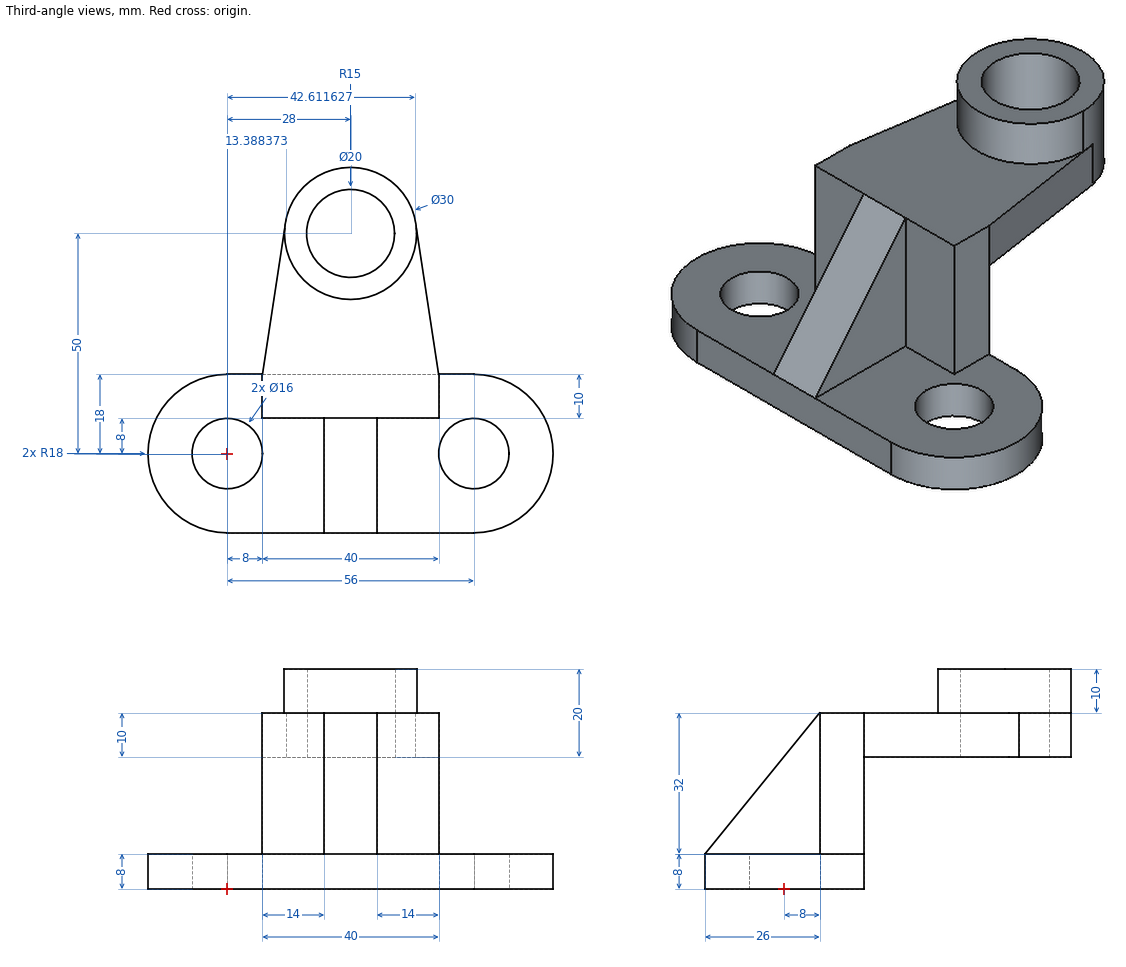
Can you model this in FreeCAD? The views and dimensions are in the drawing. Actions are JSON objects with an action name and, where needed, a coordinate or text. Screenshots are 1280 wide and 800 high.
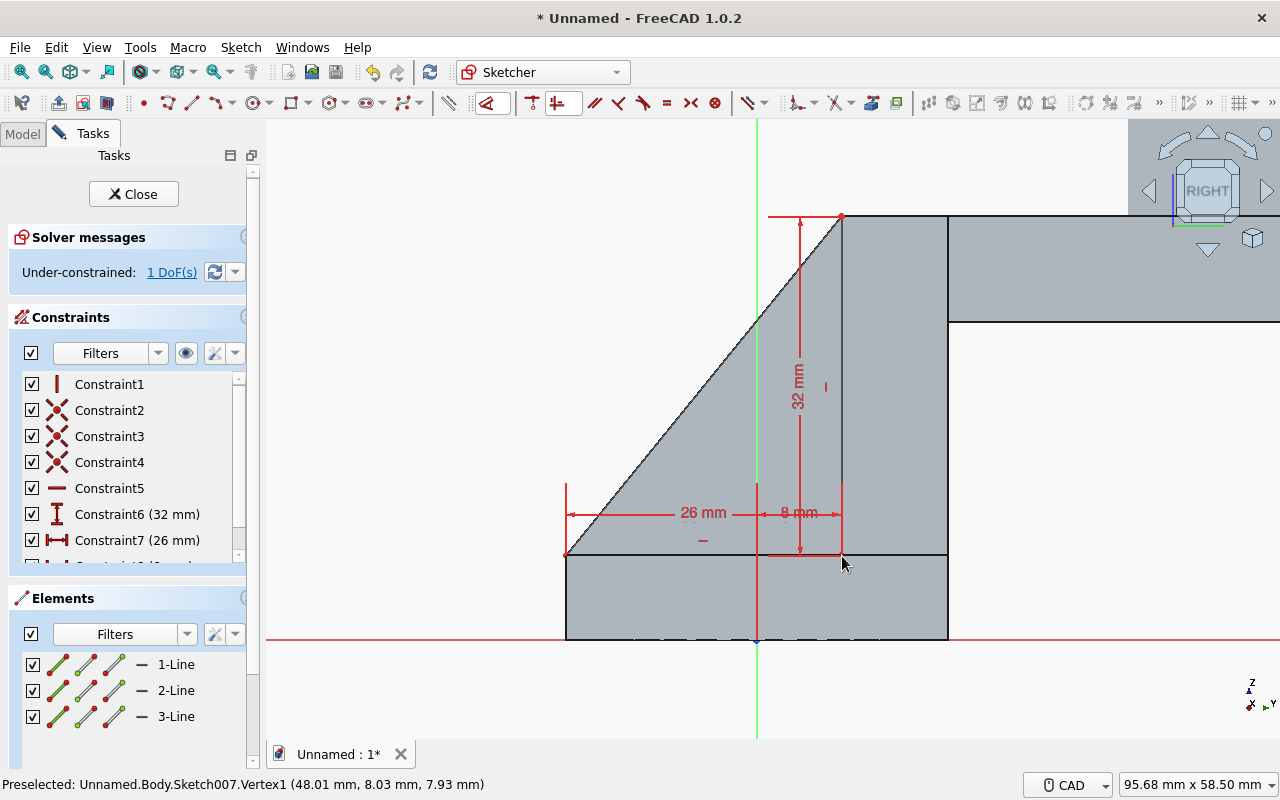
{"action": "left_click", "coordinate": [842, 556]}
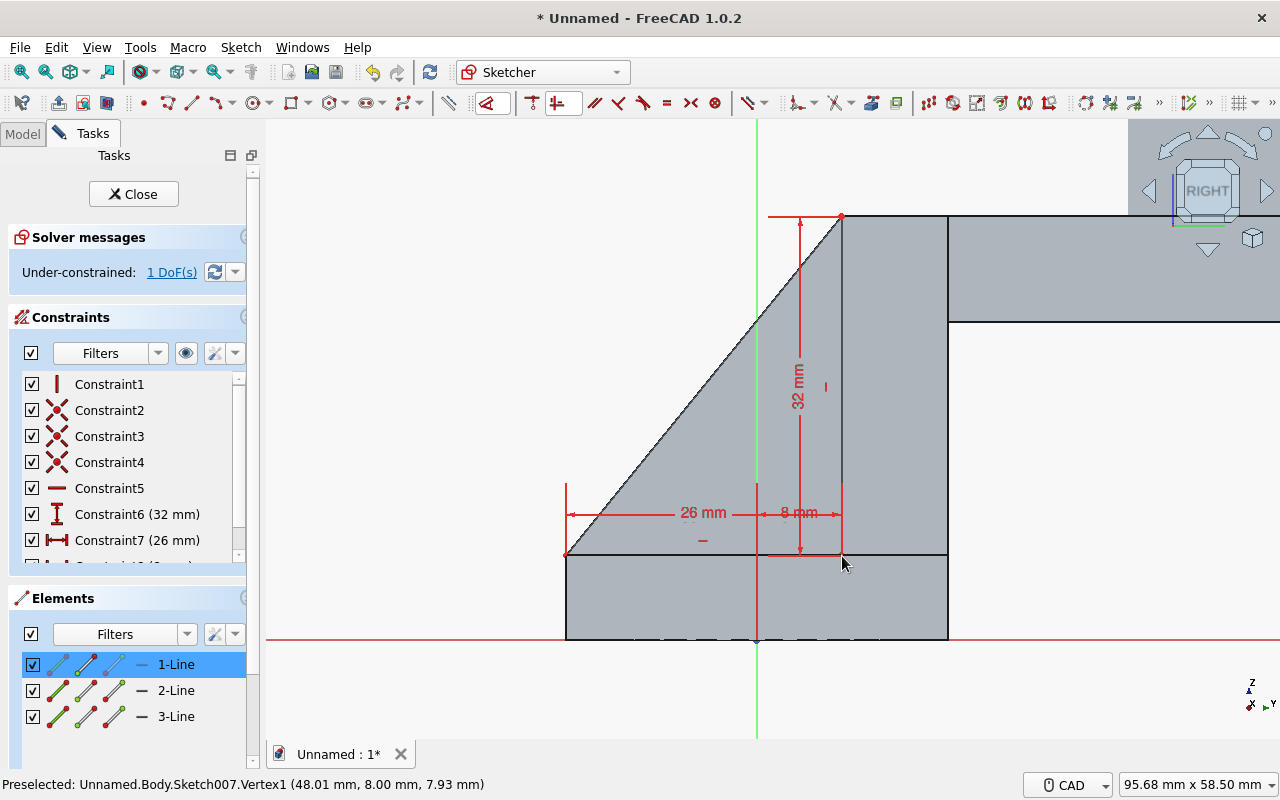
{"action": "key", "text": "i"}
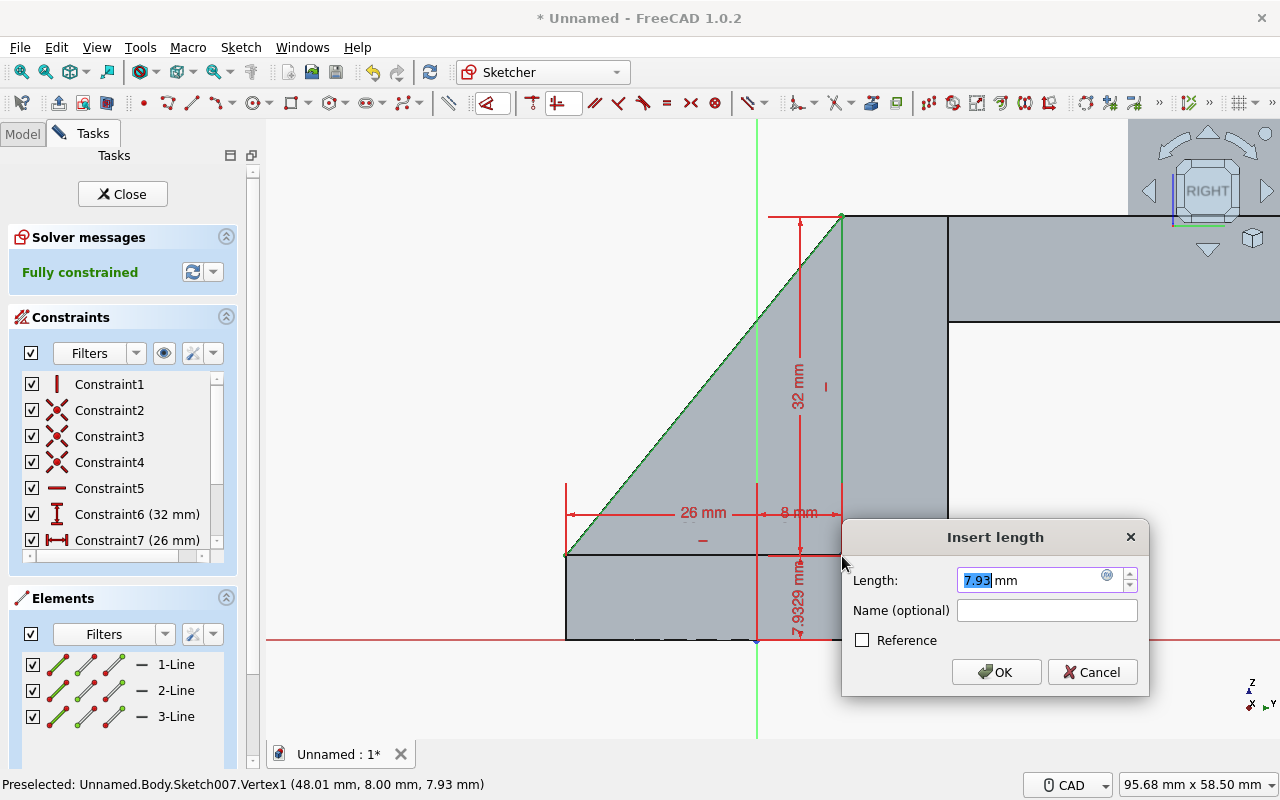
{"action": "type", "text": "8"}
{"action": "key", "text": "Return"}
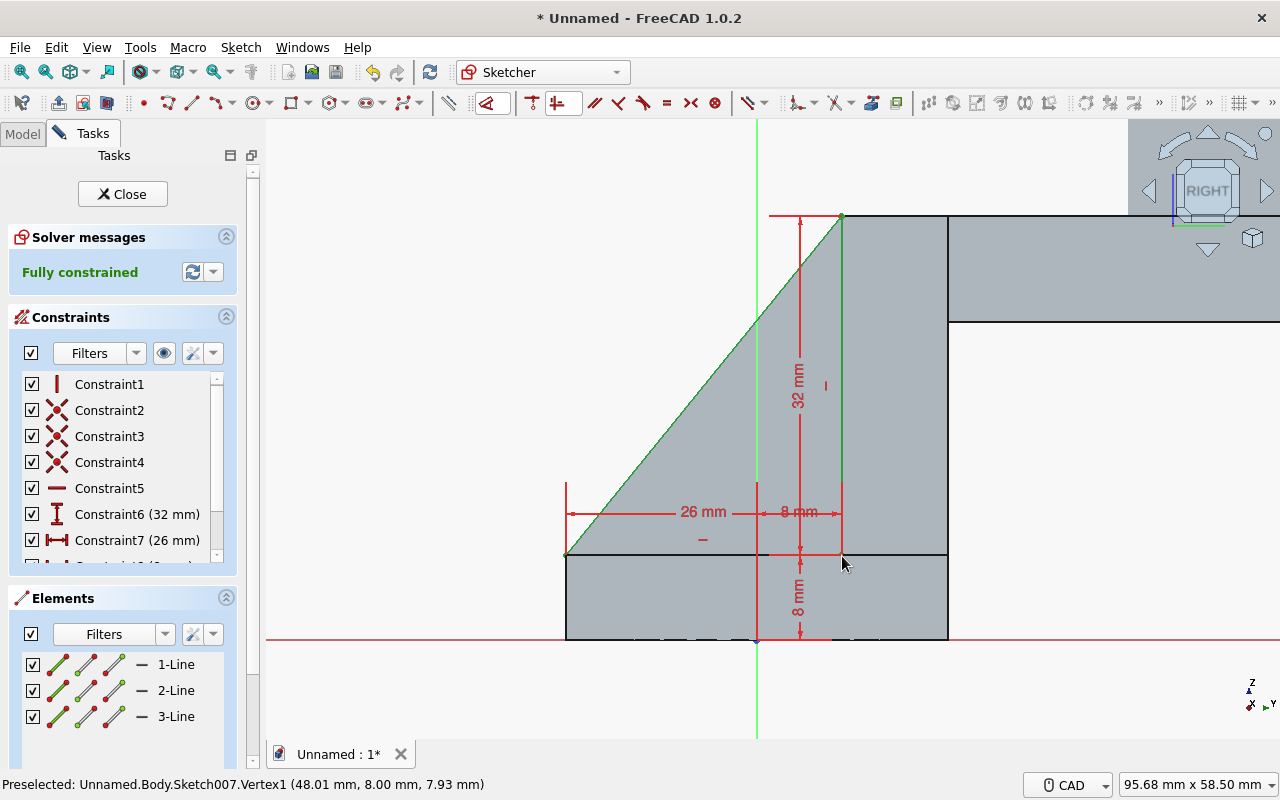
{"action": "left_click", "coordinate": [123, 194]}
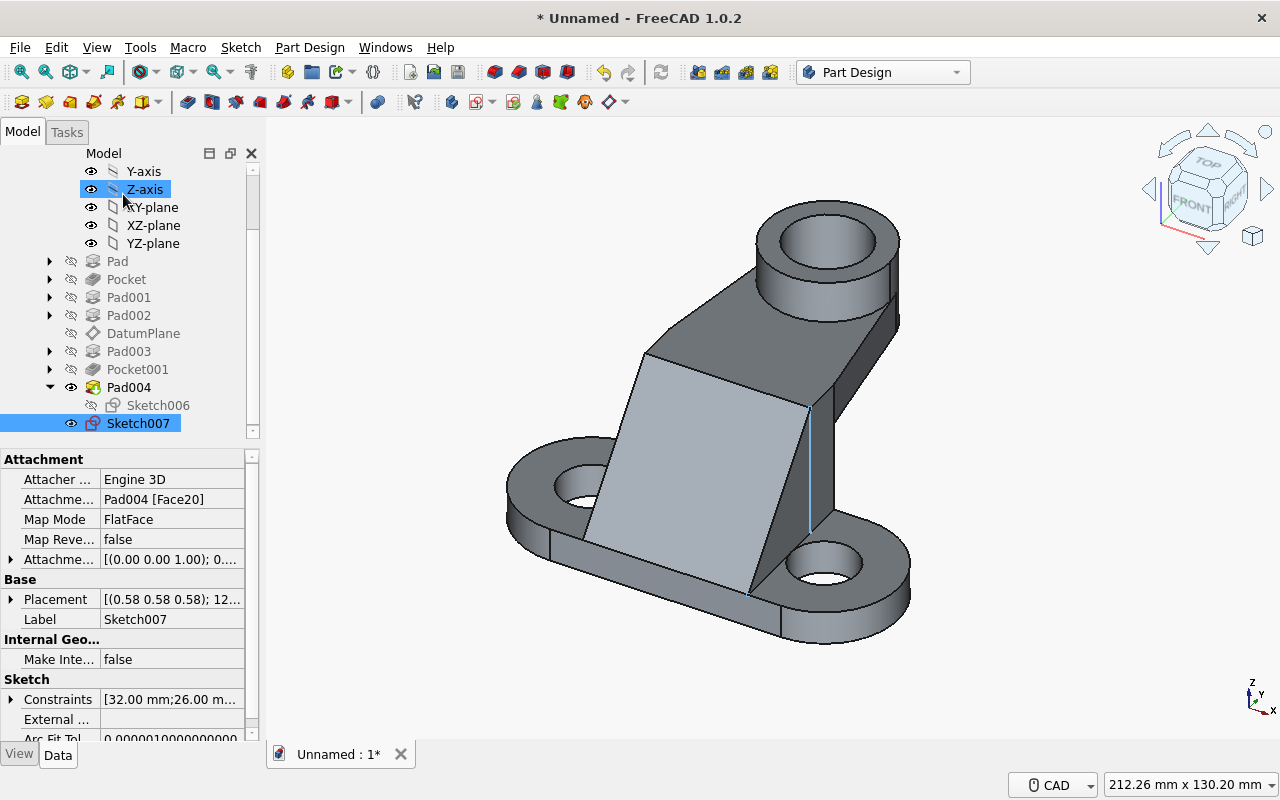
{"action": "left_click", "coordinate": [188, 102]}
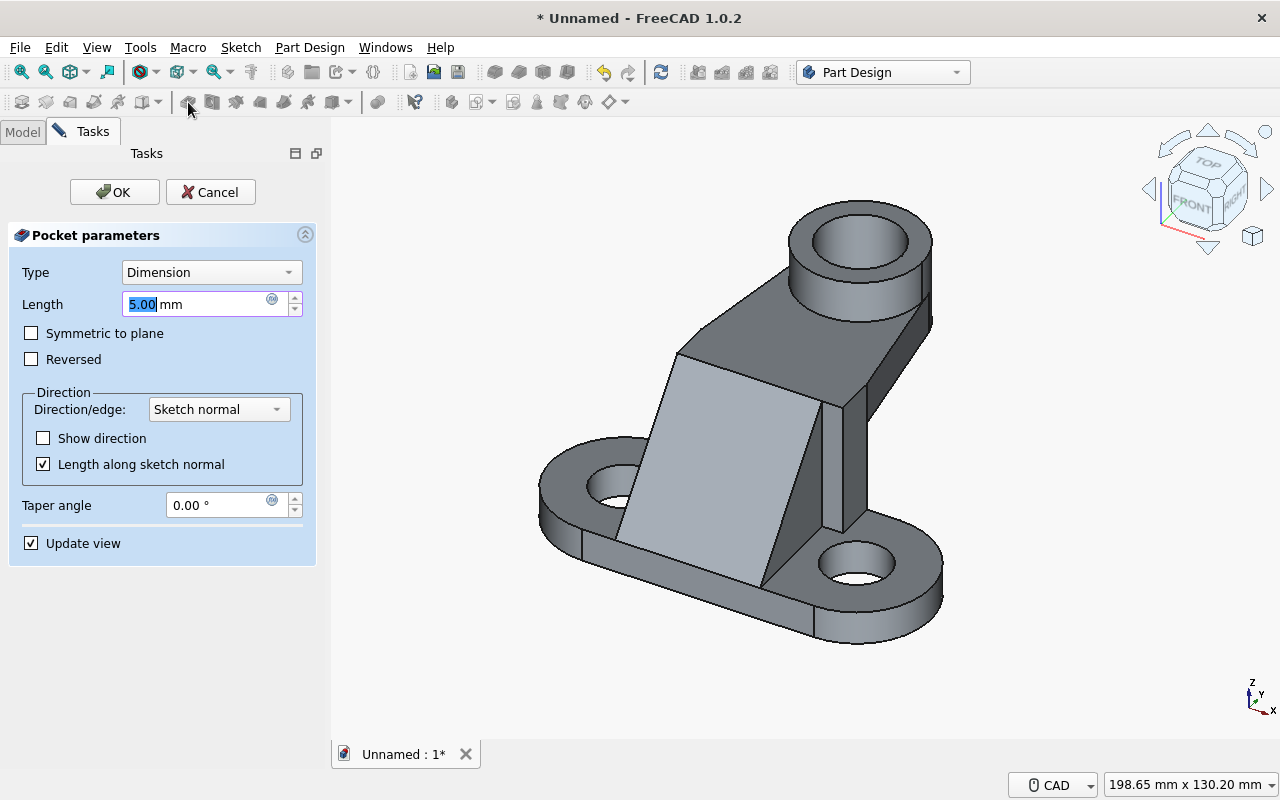
{"action": "type", "text": "14"}
{"action": "key", "text": "Tab"}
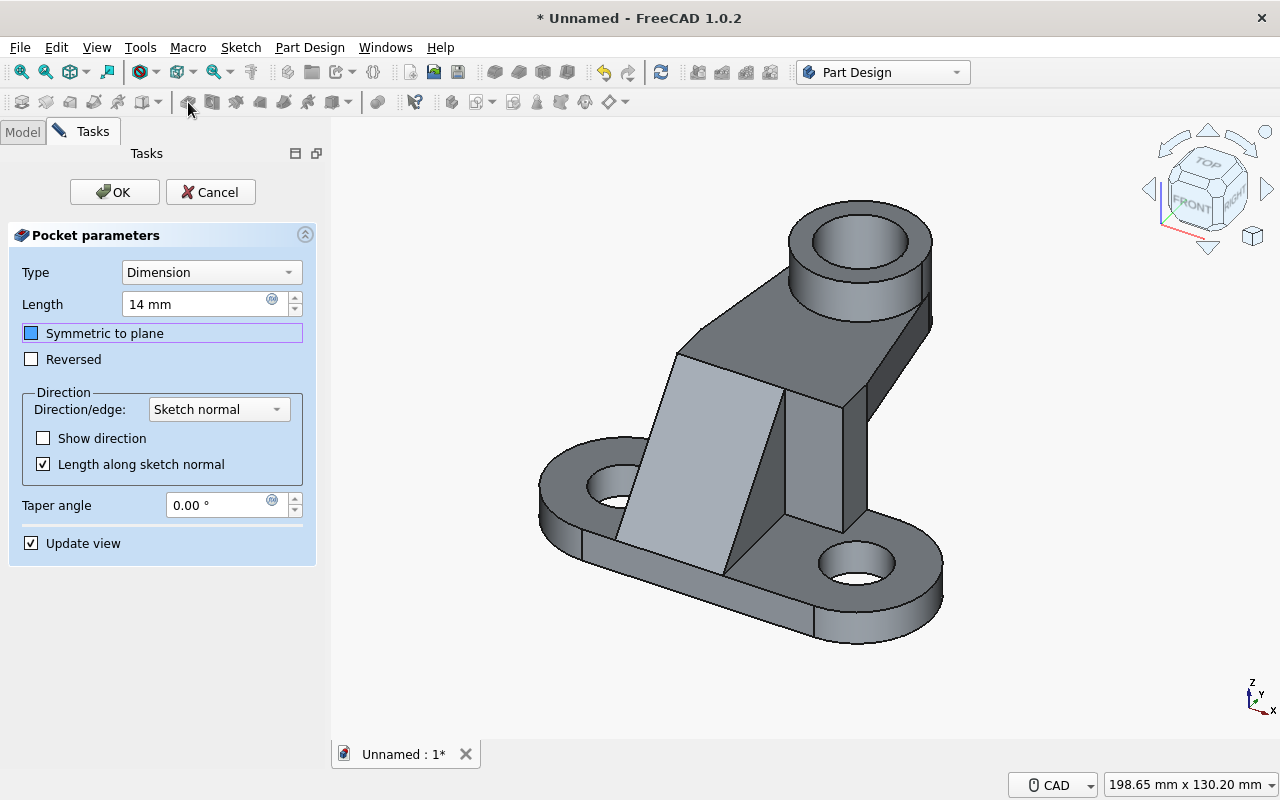
{"action": "left_click", "coordinate": [115, 192]}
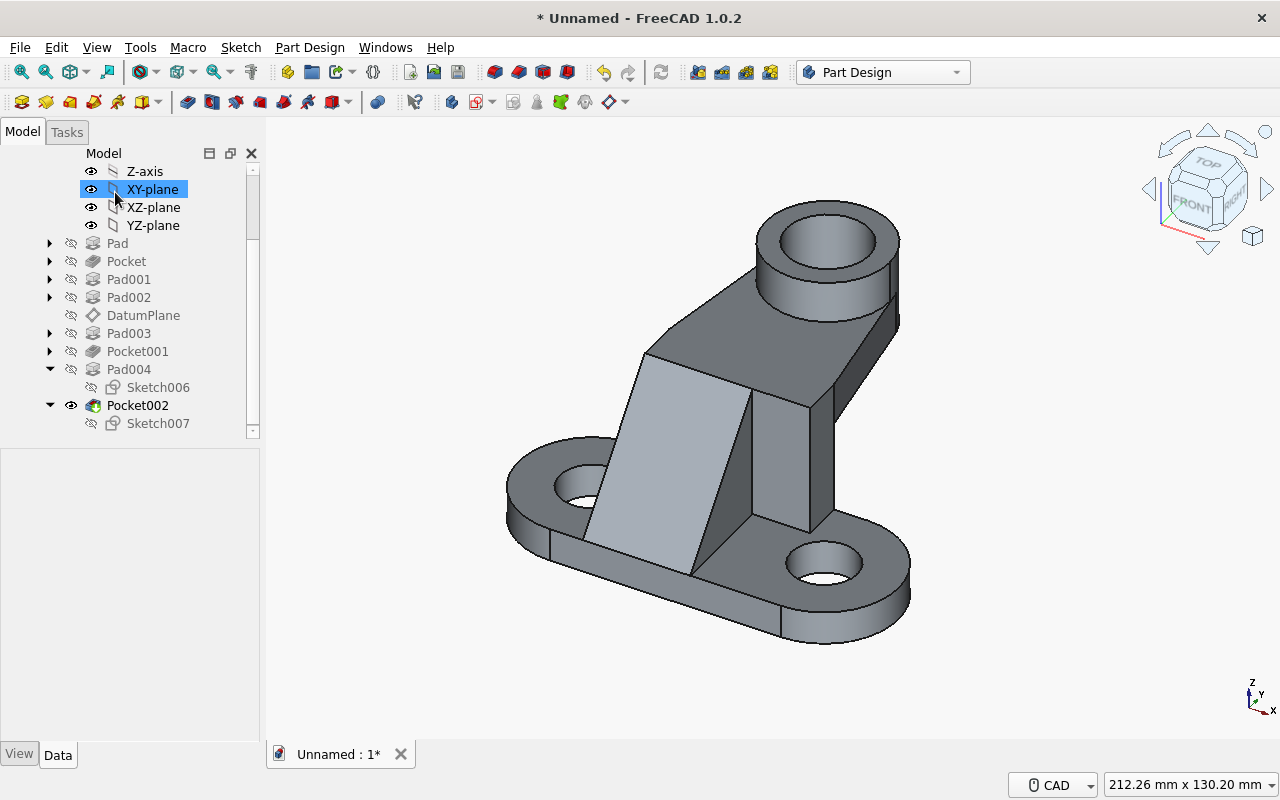
{"action": "key", "text": "6"}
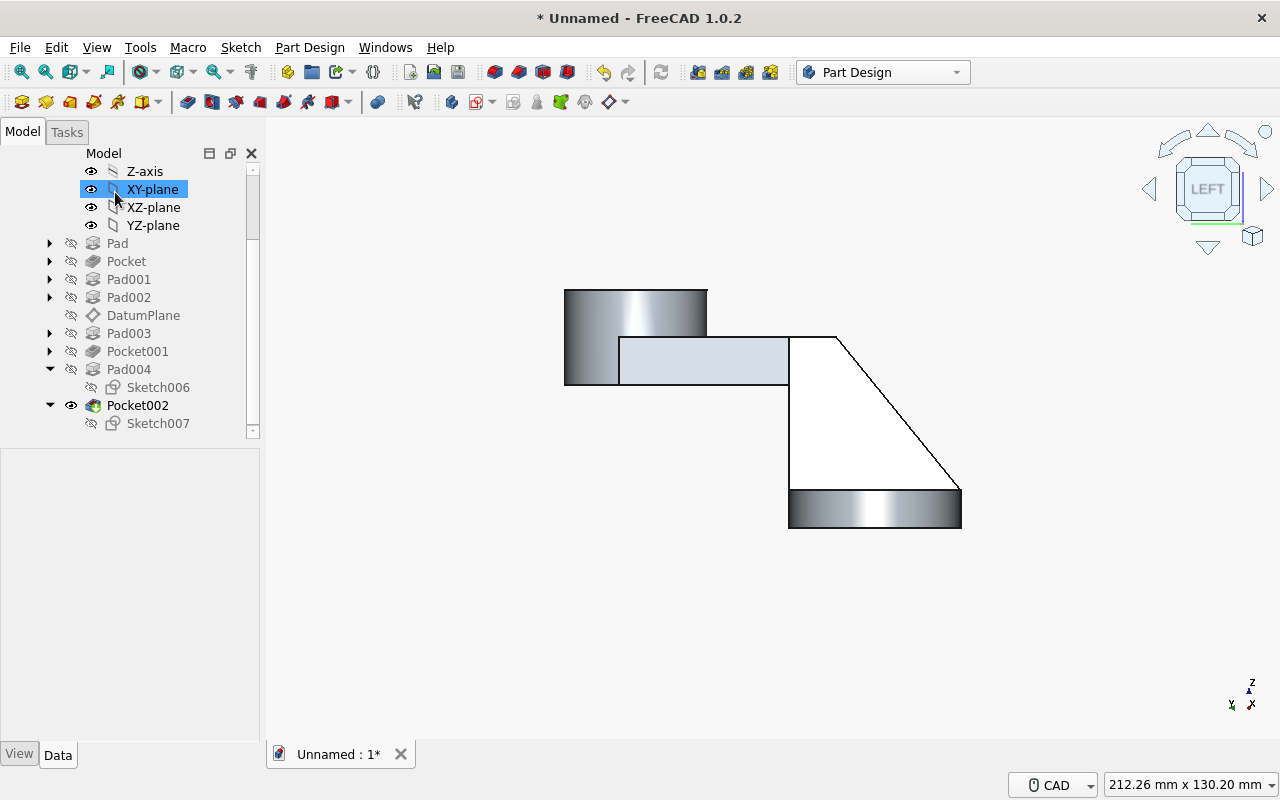
{"action": "left_click", "coordinate": [22, 72]}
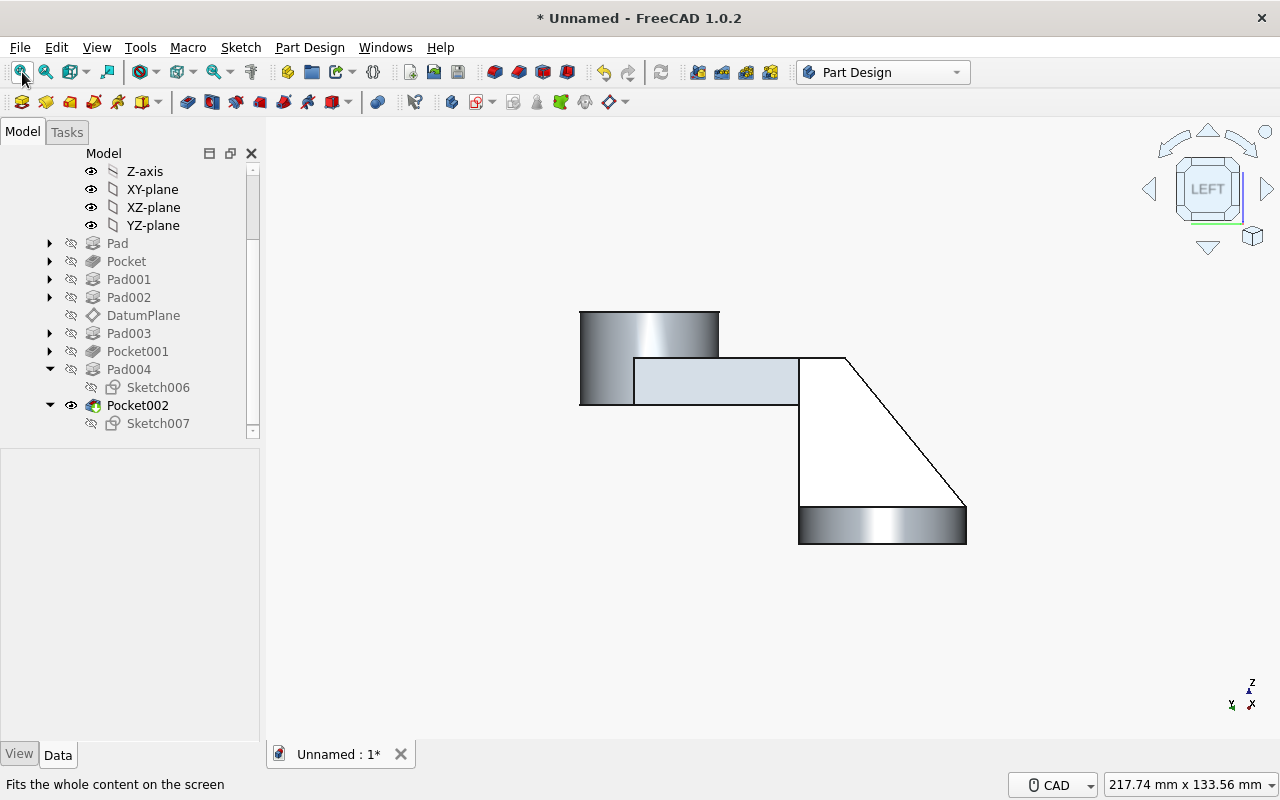
{"action": "left_click", "coordinate": [858, 453]}